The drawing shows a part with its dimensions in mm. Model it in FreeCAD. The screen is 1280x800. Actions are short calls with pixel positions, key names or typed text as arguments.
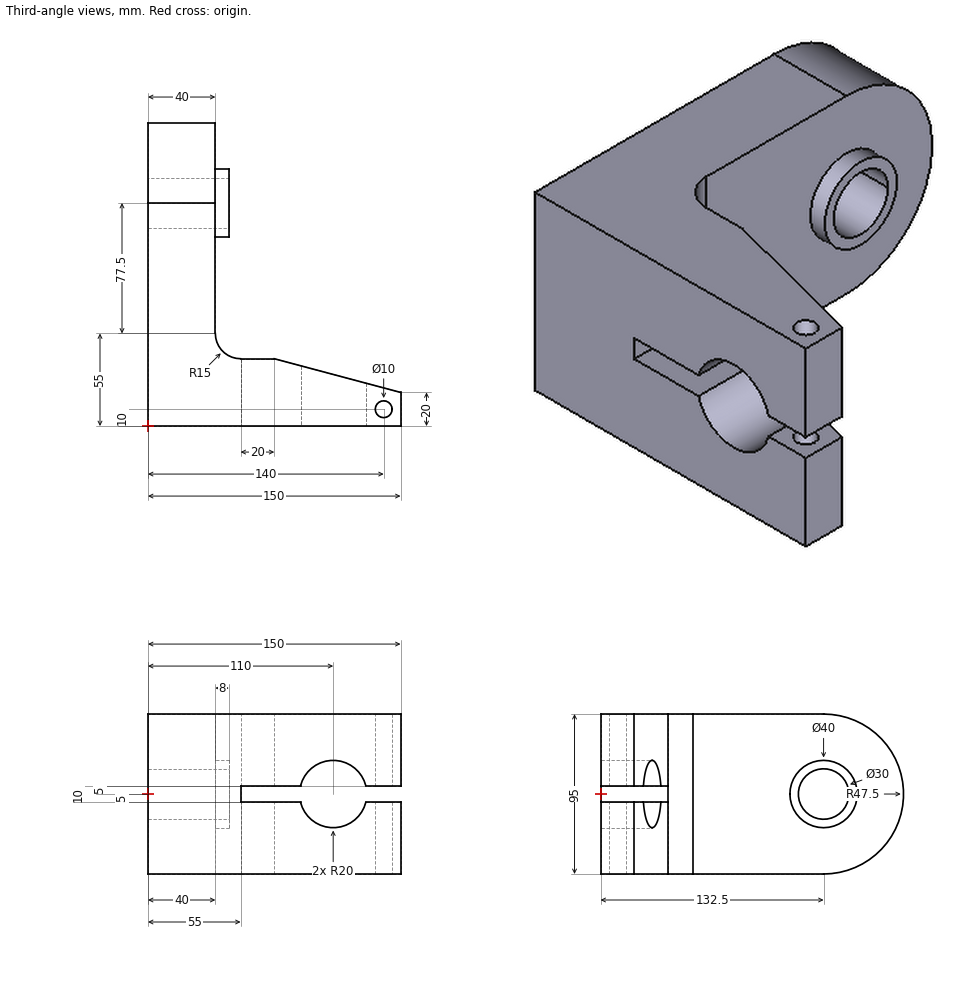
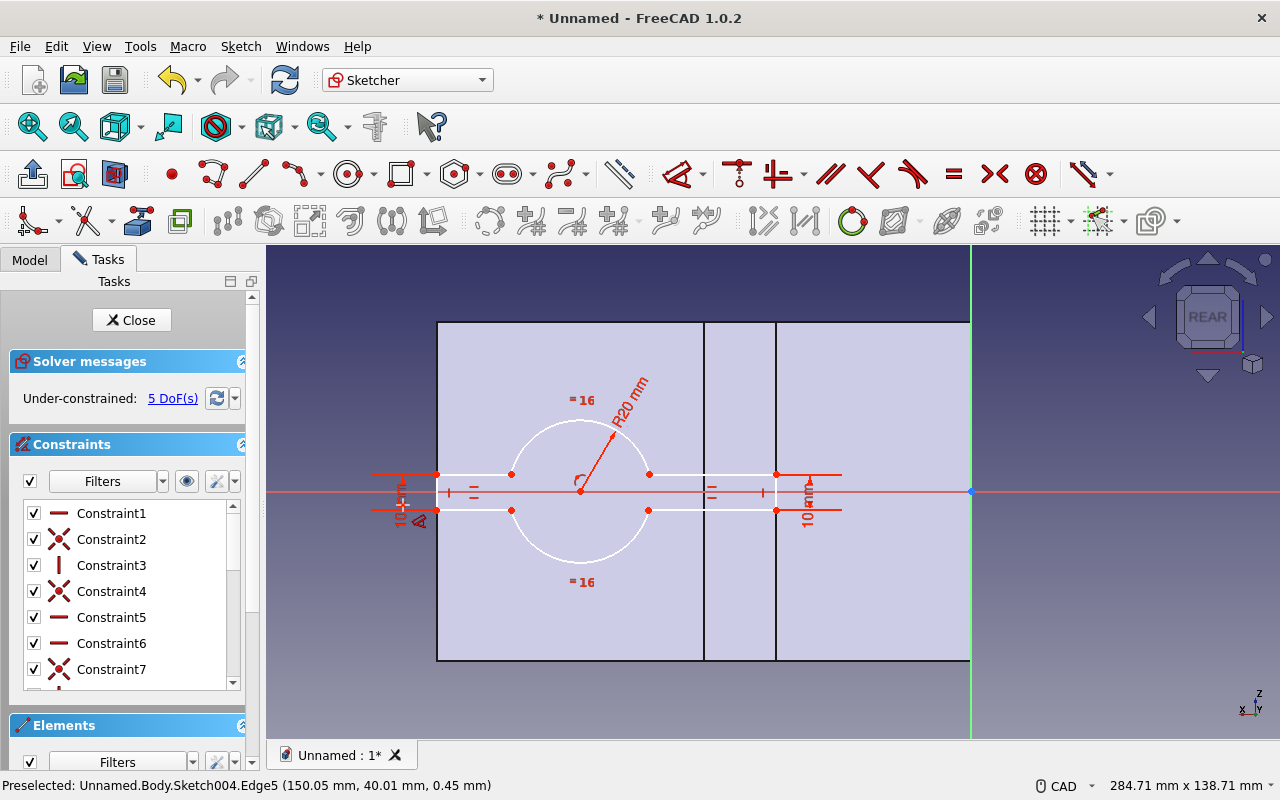
scroll(649, 510, up, 5)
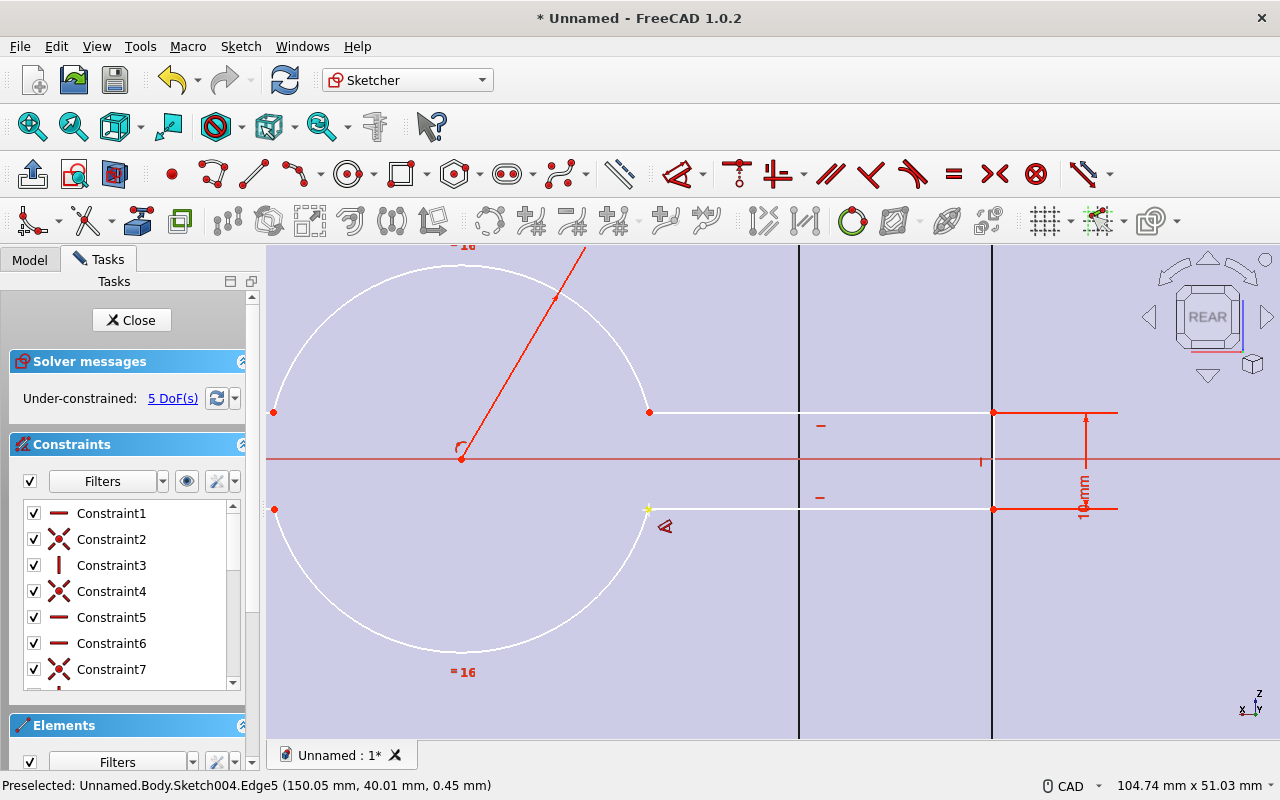
click(648, 509)
click(614, 484)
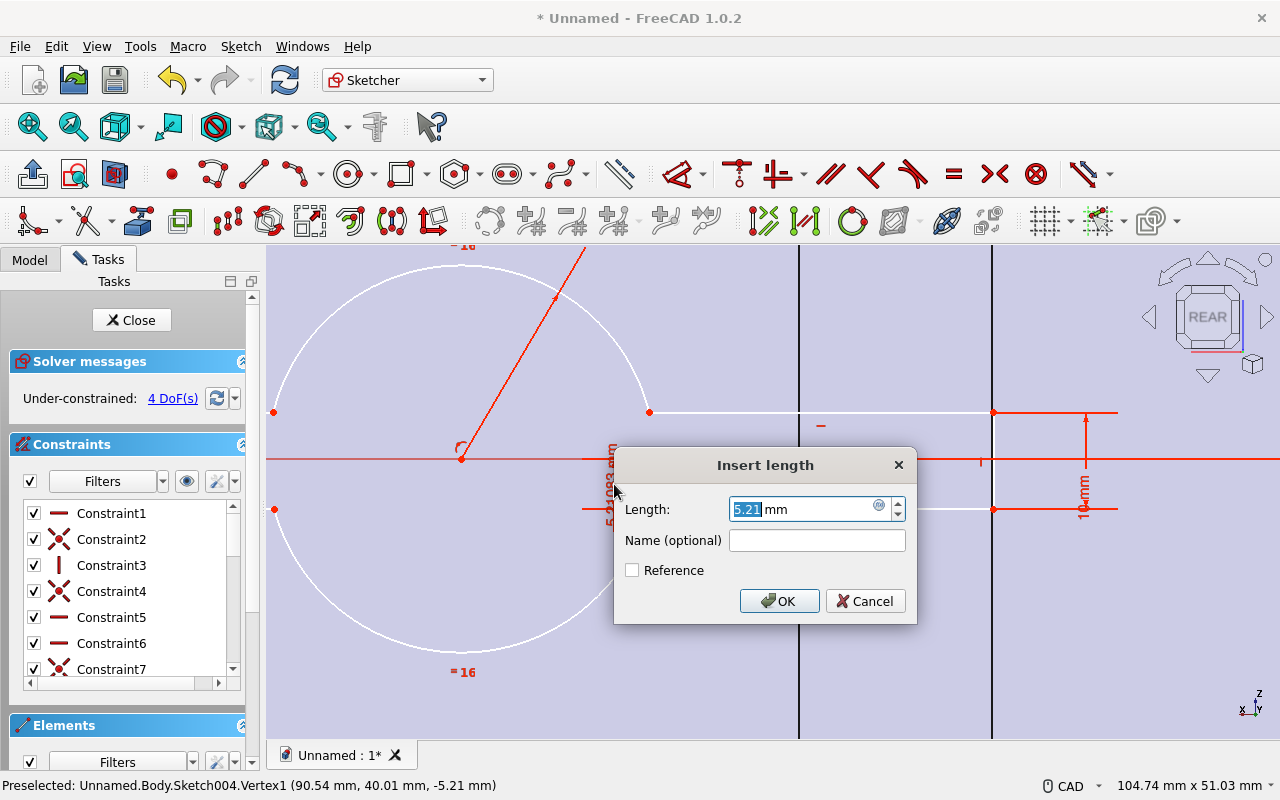
text(5)
key(Return)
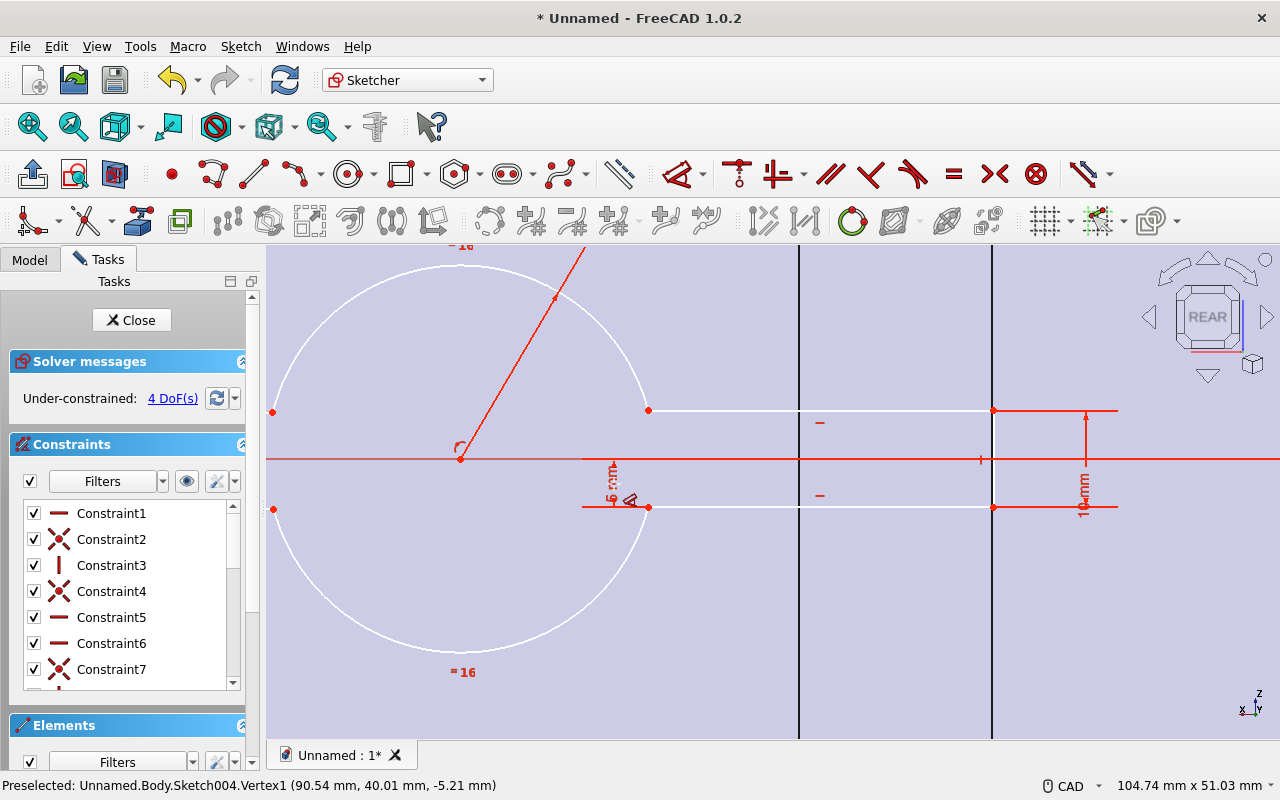
scroll(650, 511, down, 5)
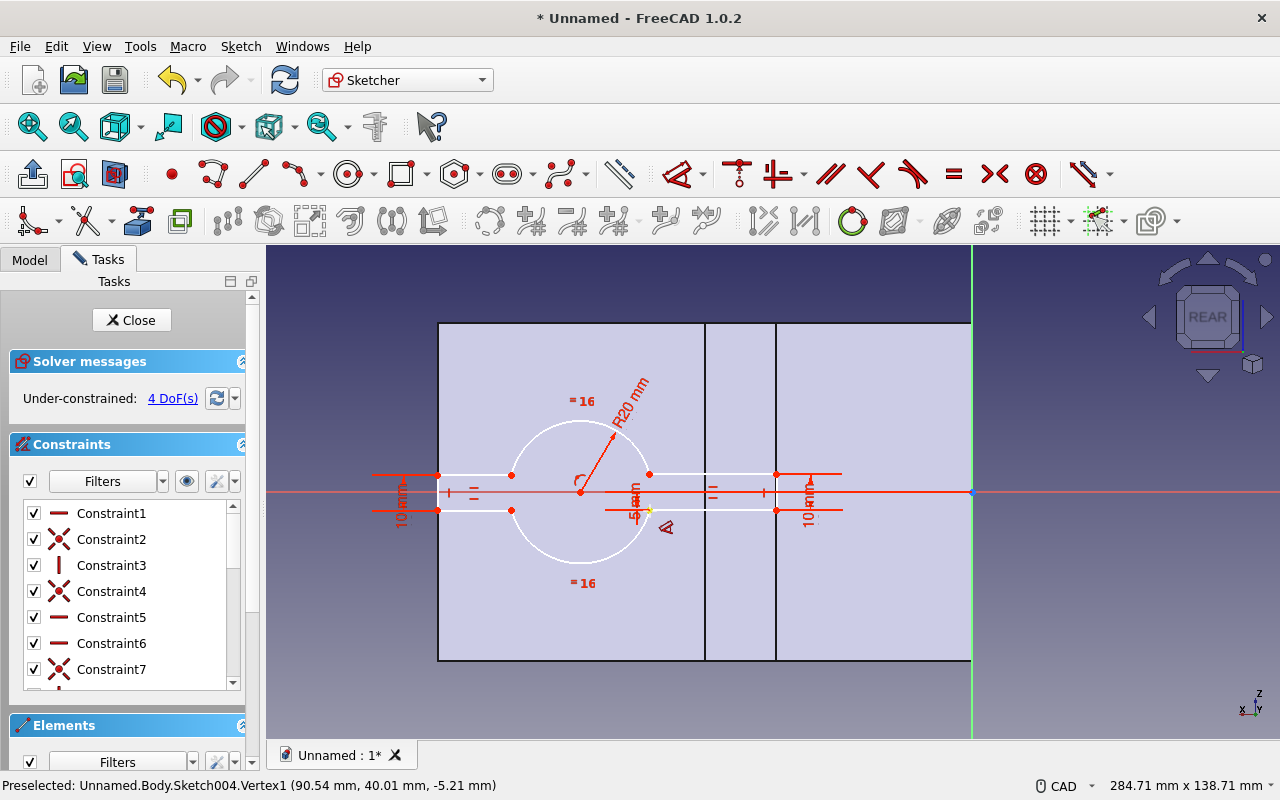
scroll(511, 475, up, 5)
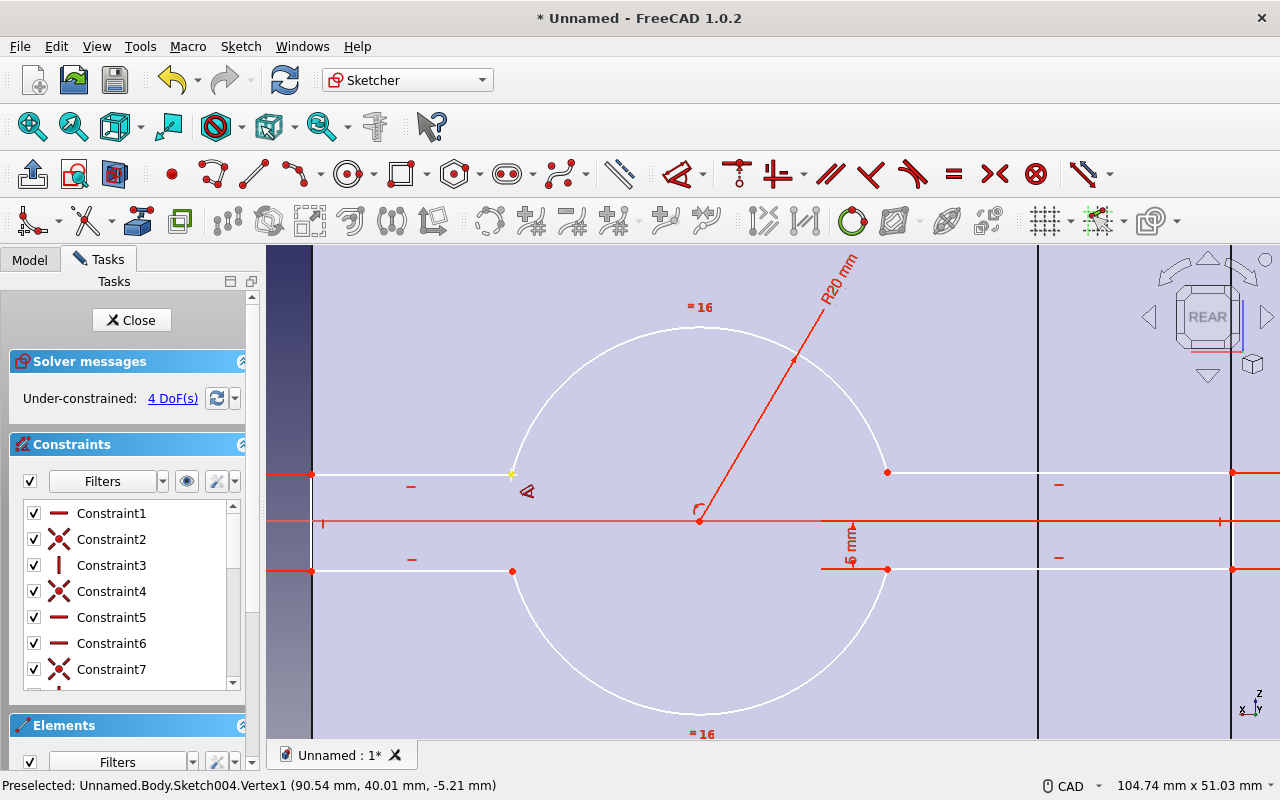
click(512, 475)
click(478, 498)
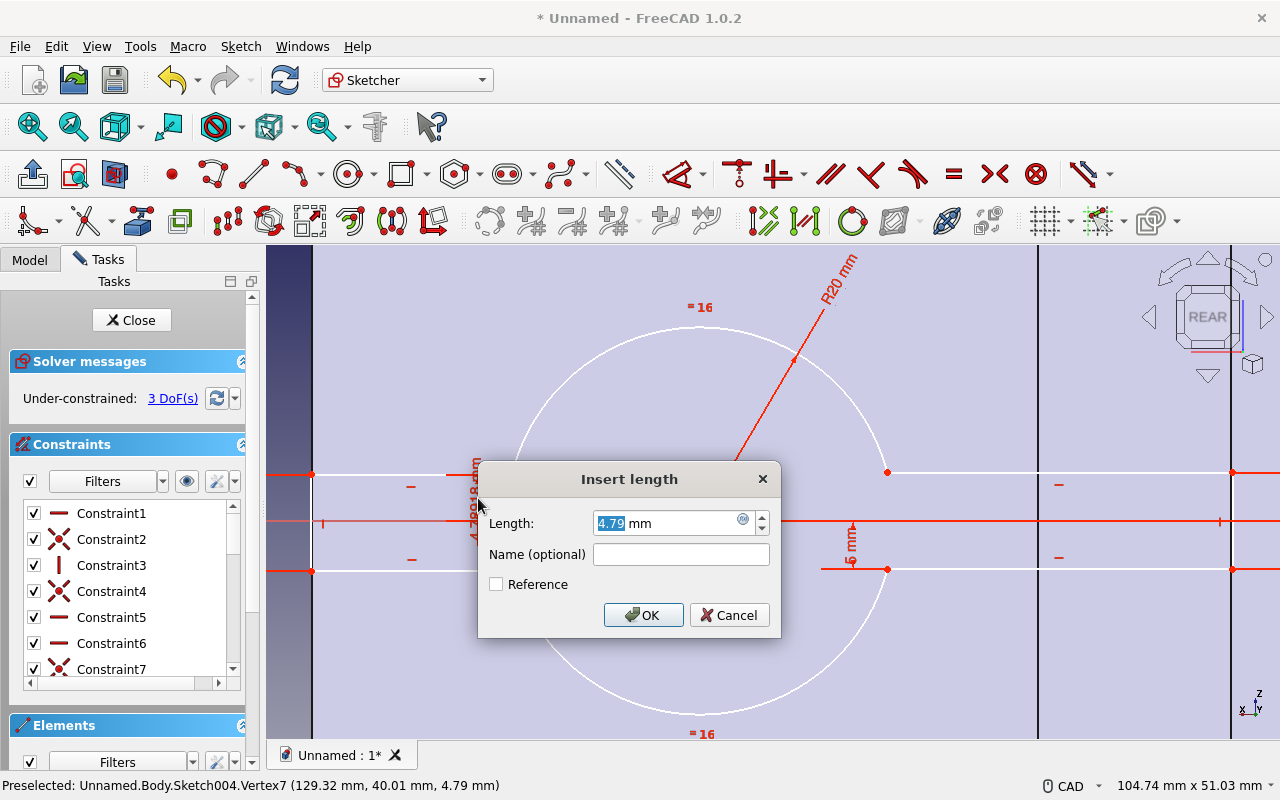
text(5)
key(Return)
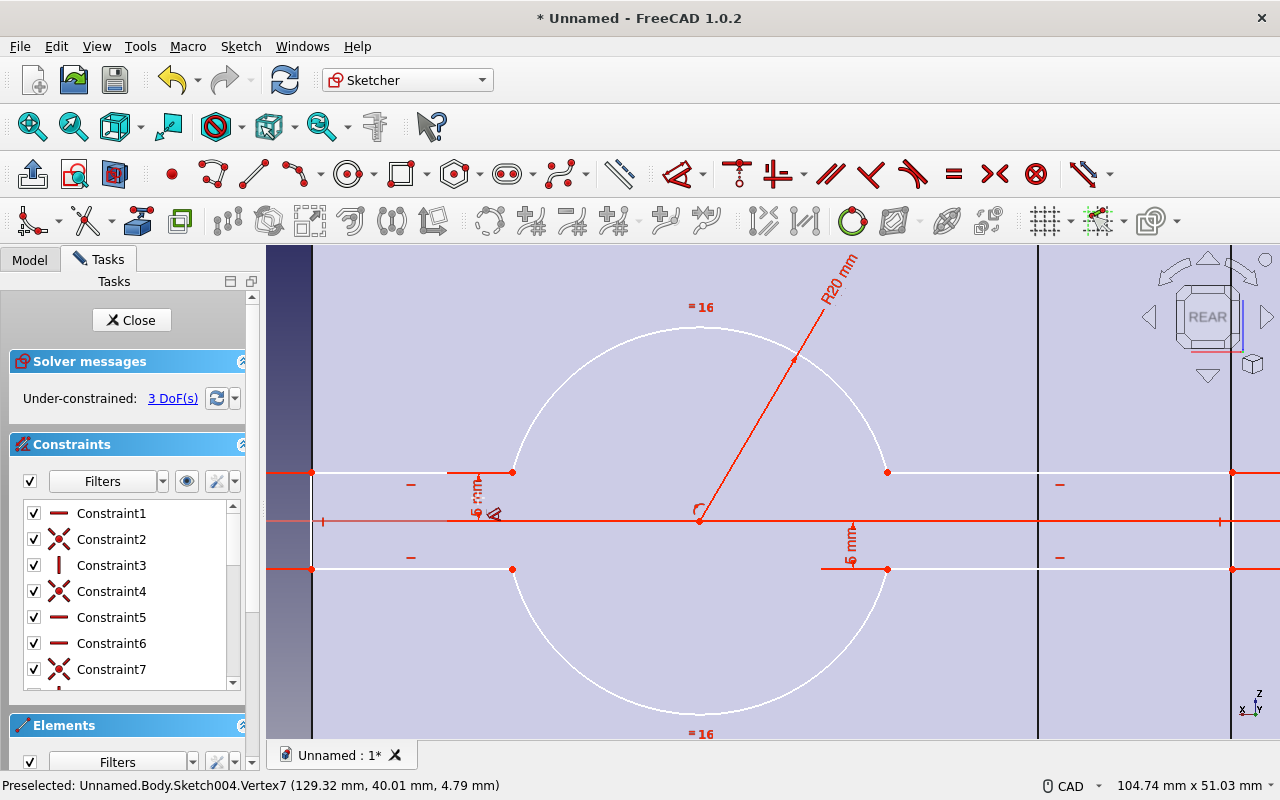
scroll(511, 475, down, 5)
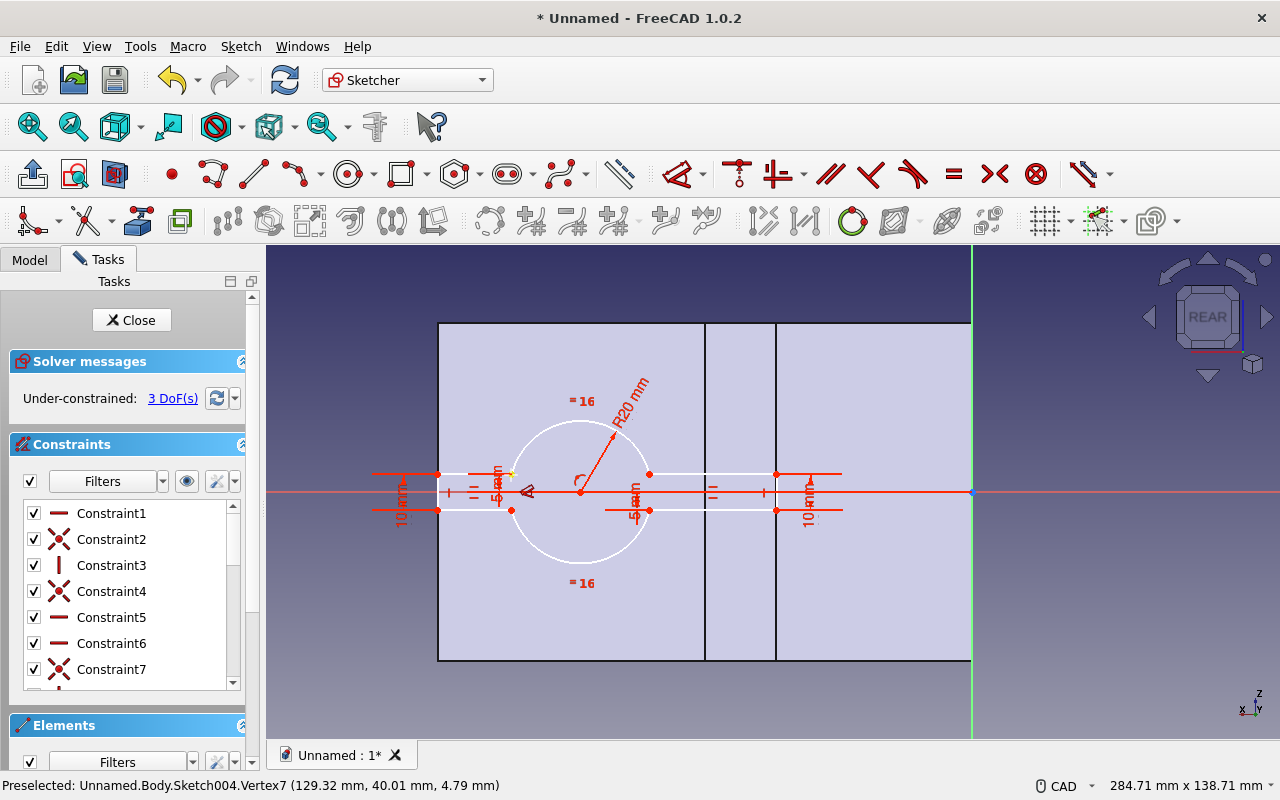
click(777, 510)
click(874, 544)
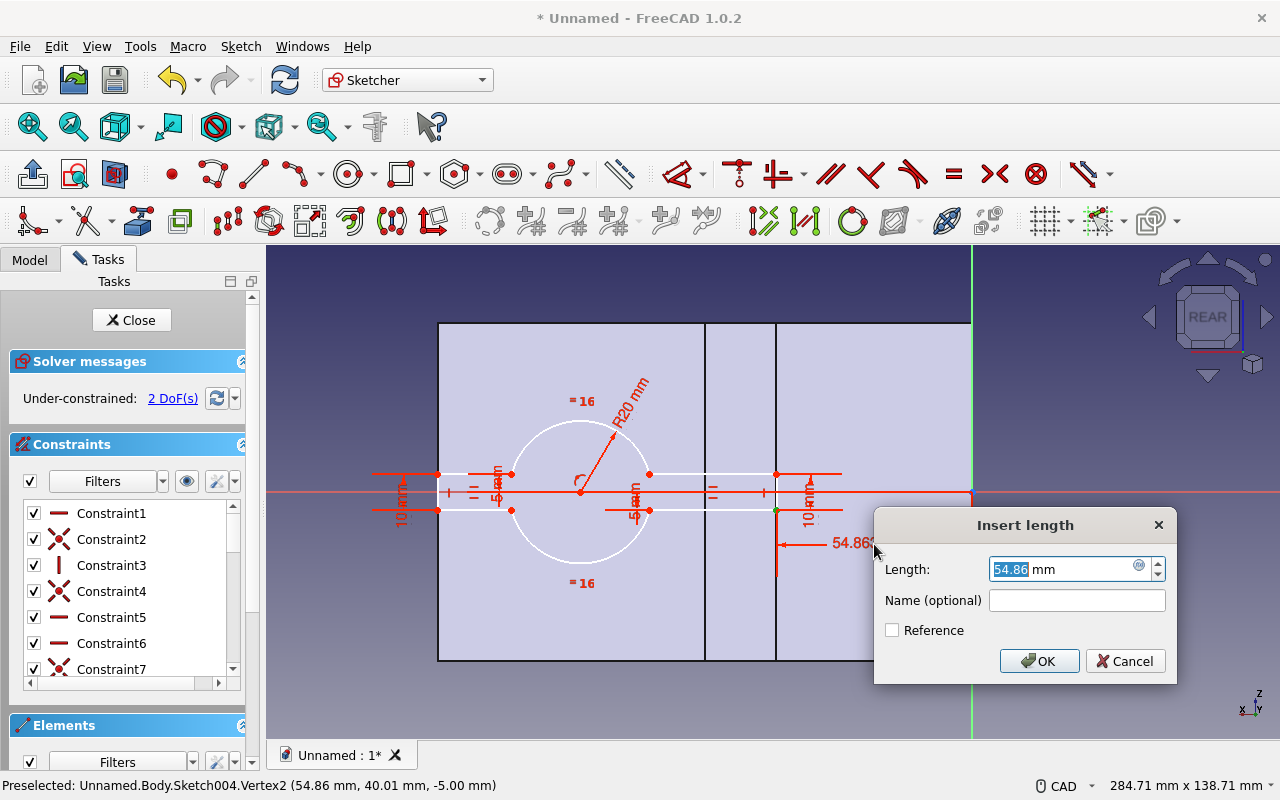
text(55)
key(Return)